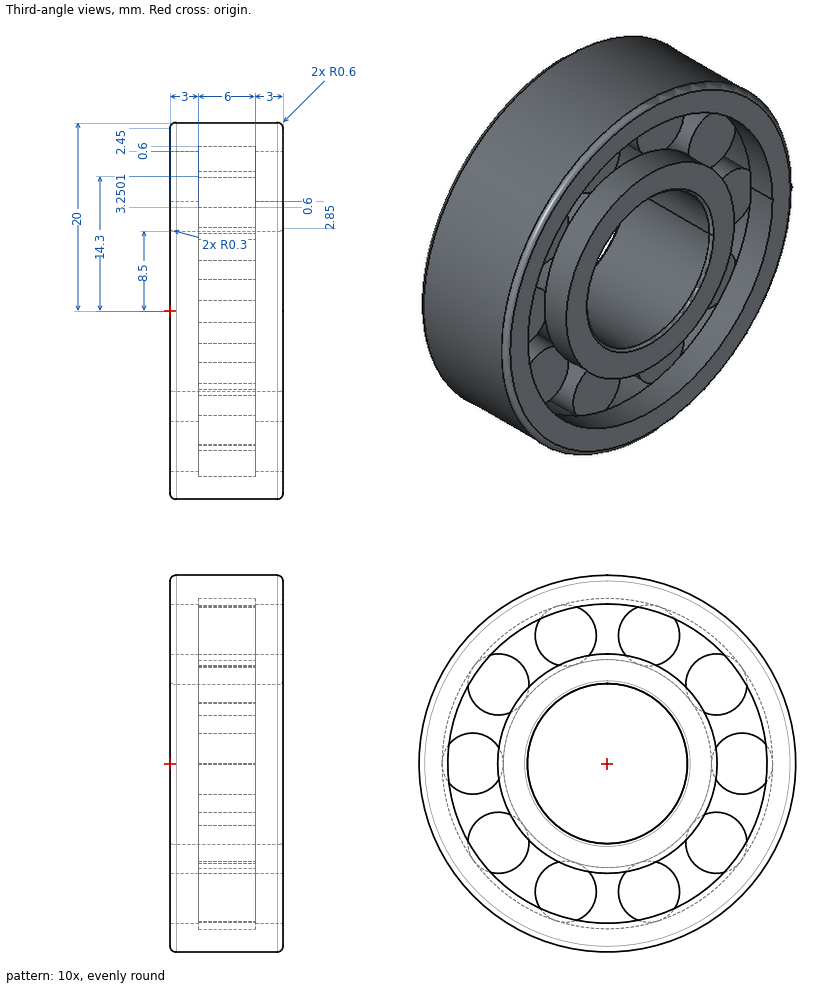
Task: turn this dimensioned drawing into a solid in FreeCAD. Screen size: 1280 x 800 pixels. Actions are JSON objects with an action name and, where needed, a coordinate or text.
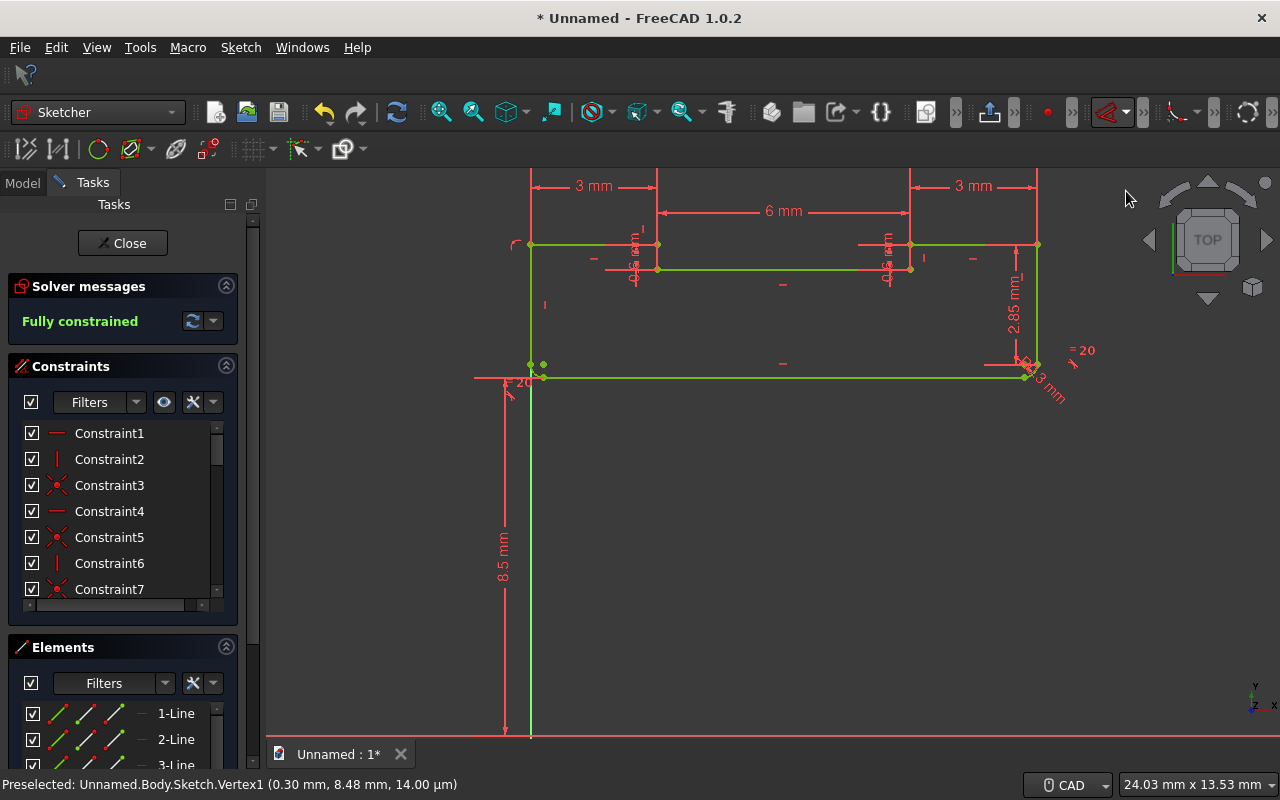
{"action": "left_click", "coordinate": [123, 243]}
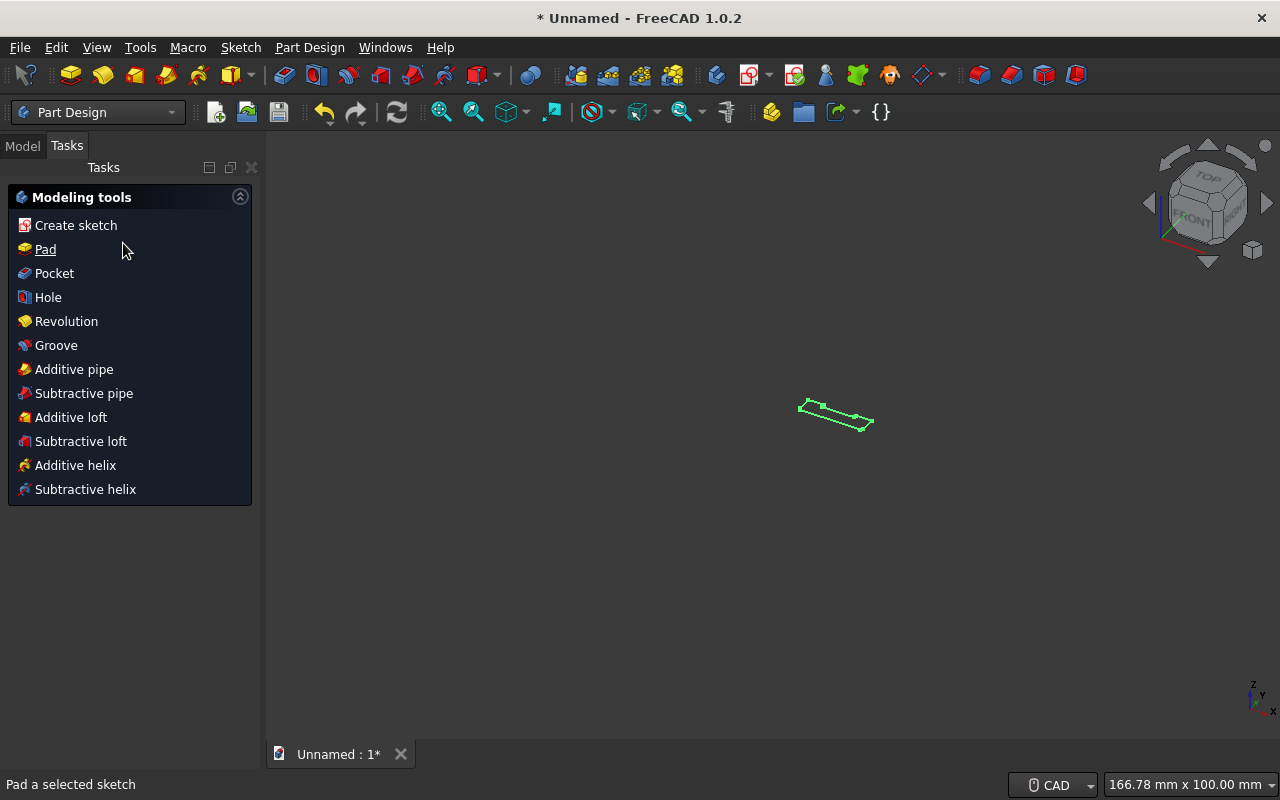
{"action": "left_click", "coordinate": [104, 76]}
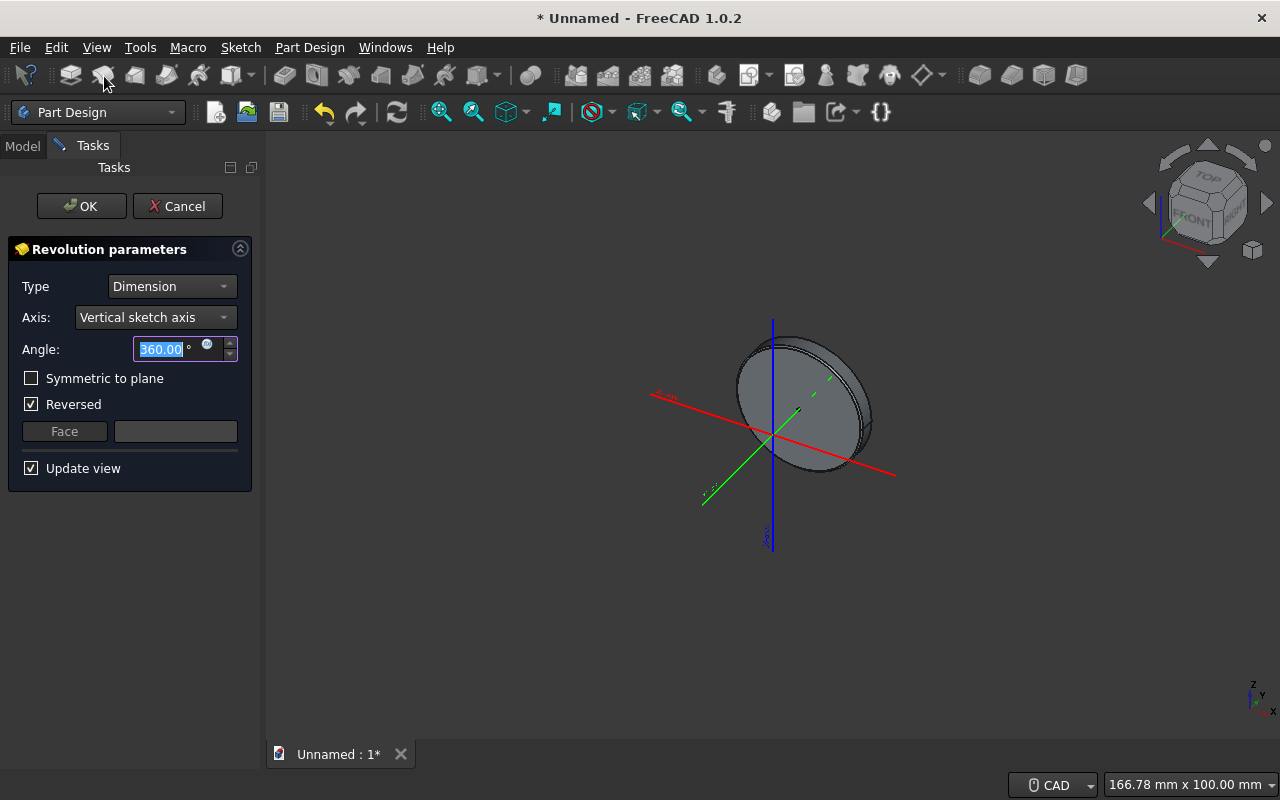
{"action": "left_click", "coordinate": [156, 318]}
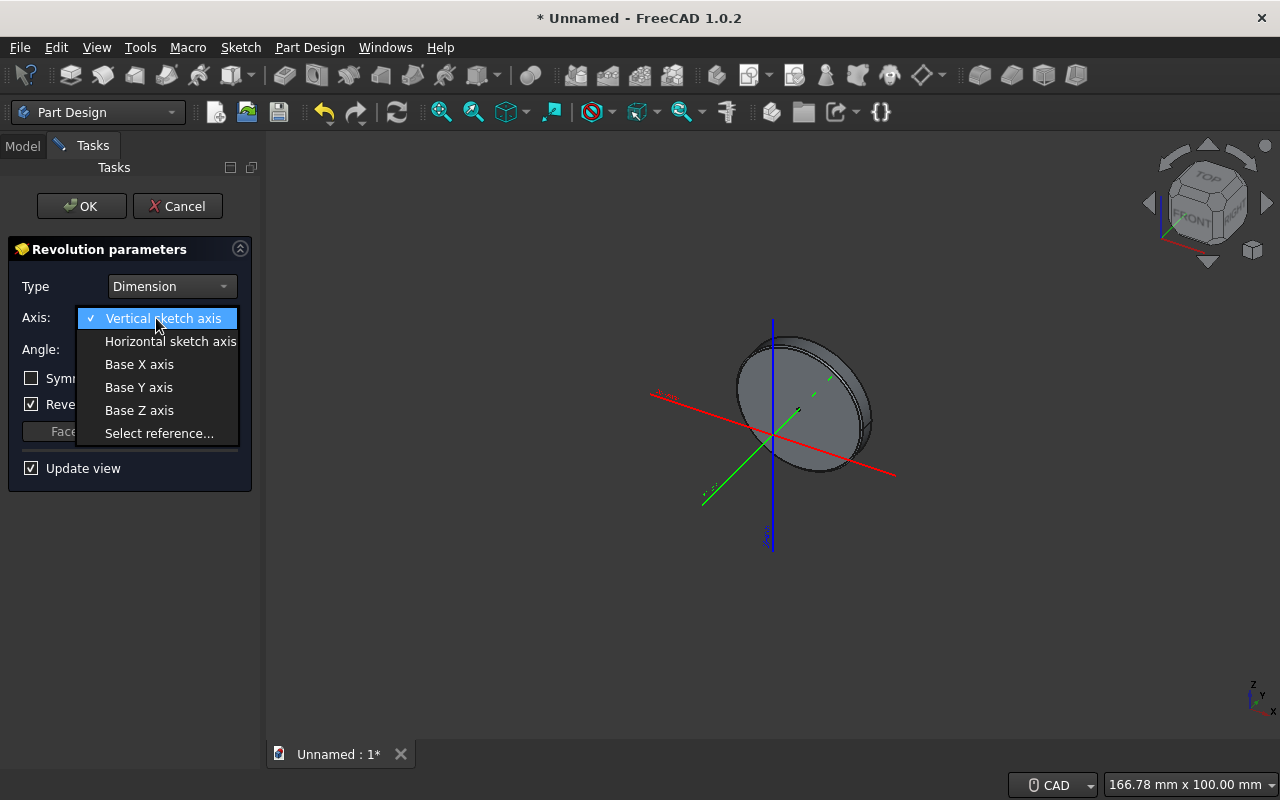
{"action": "left_click", "coordinate": [156, 342]}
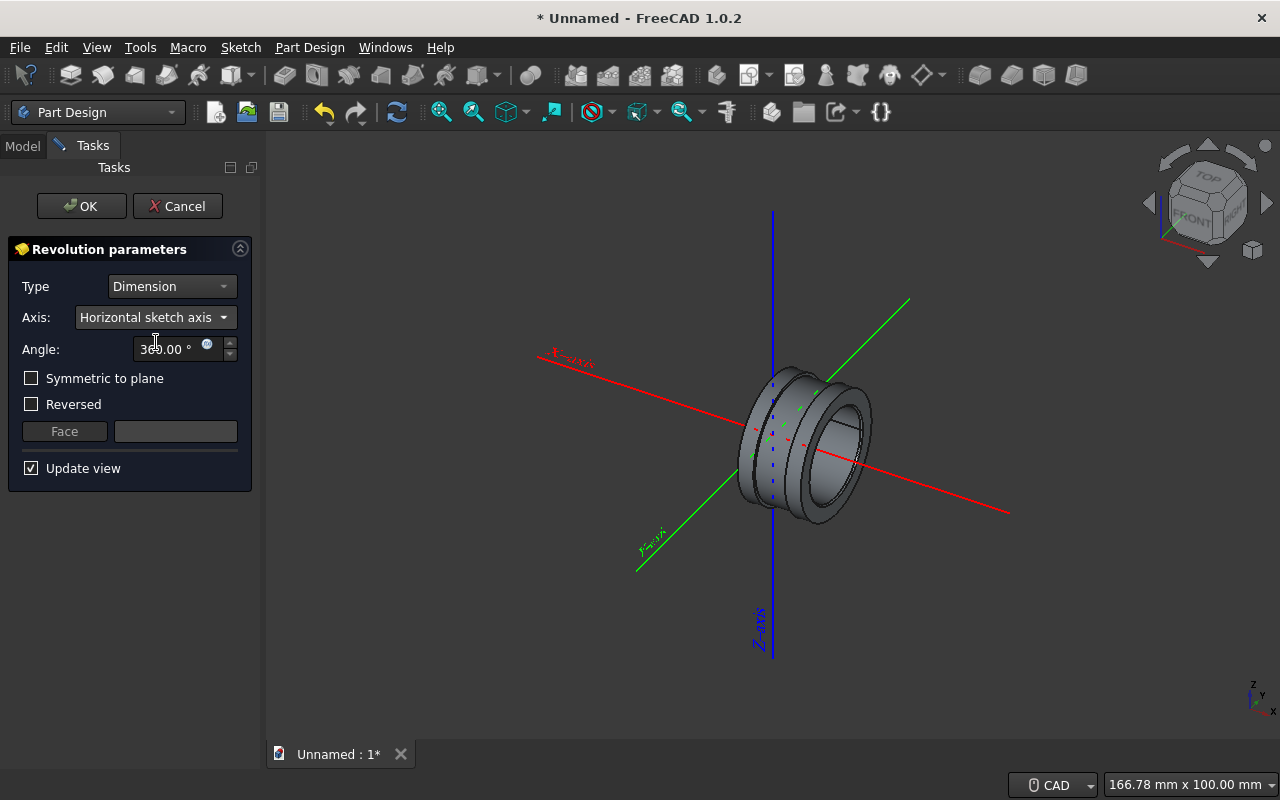
{"action": "left_click", "coordinate": [82, 206]}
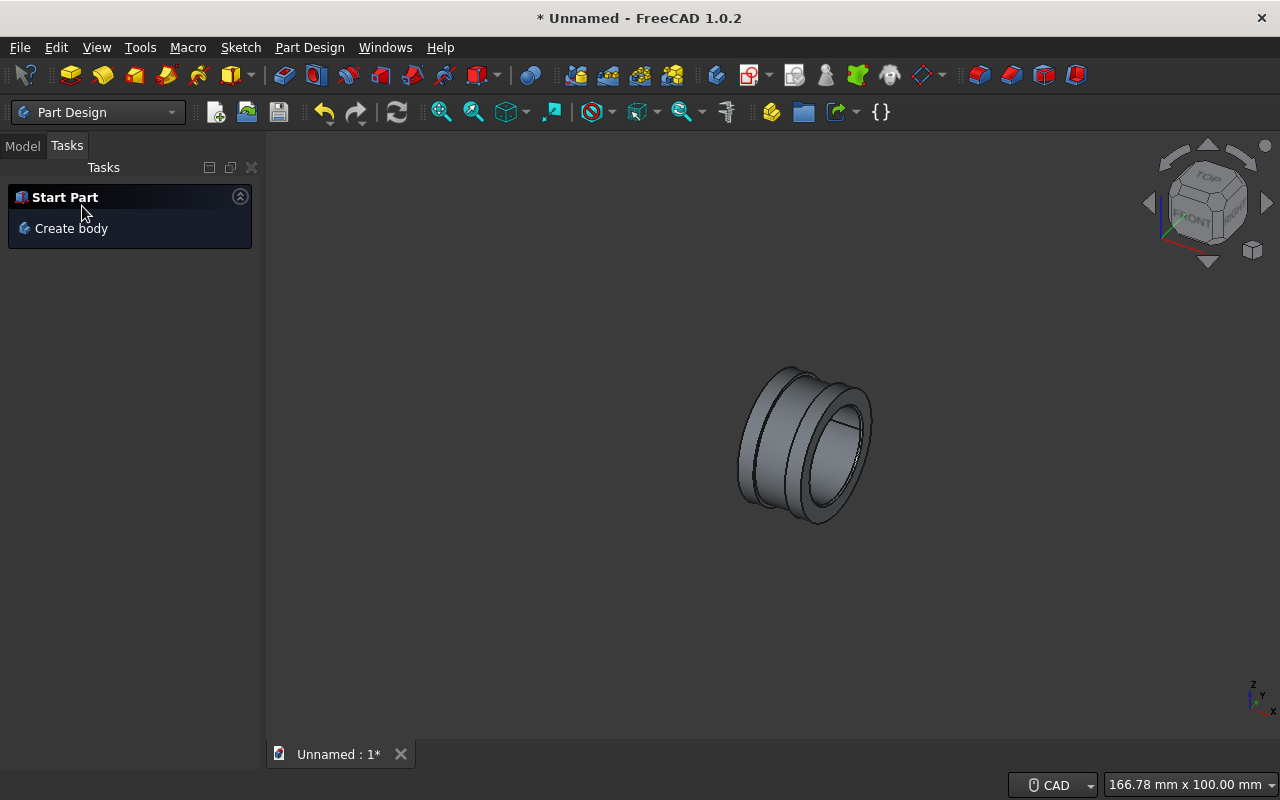
{"action": "left_click", "coordinate": [442, 112]}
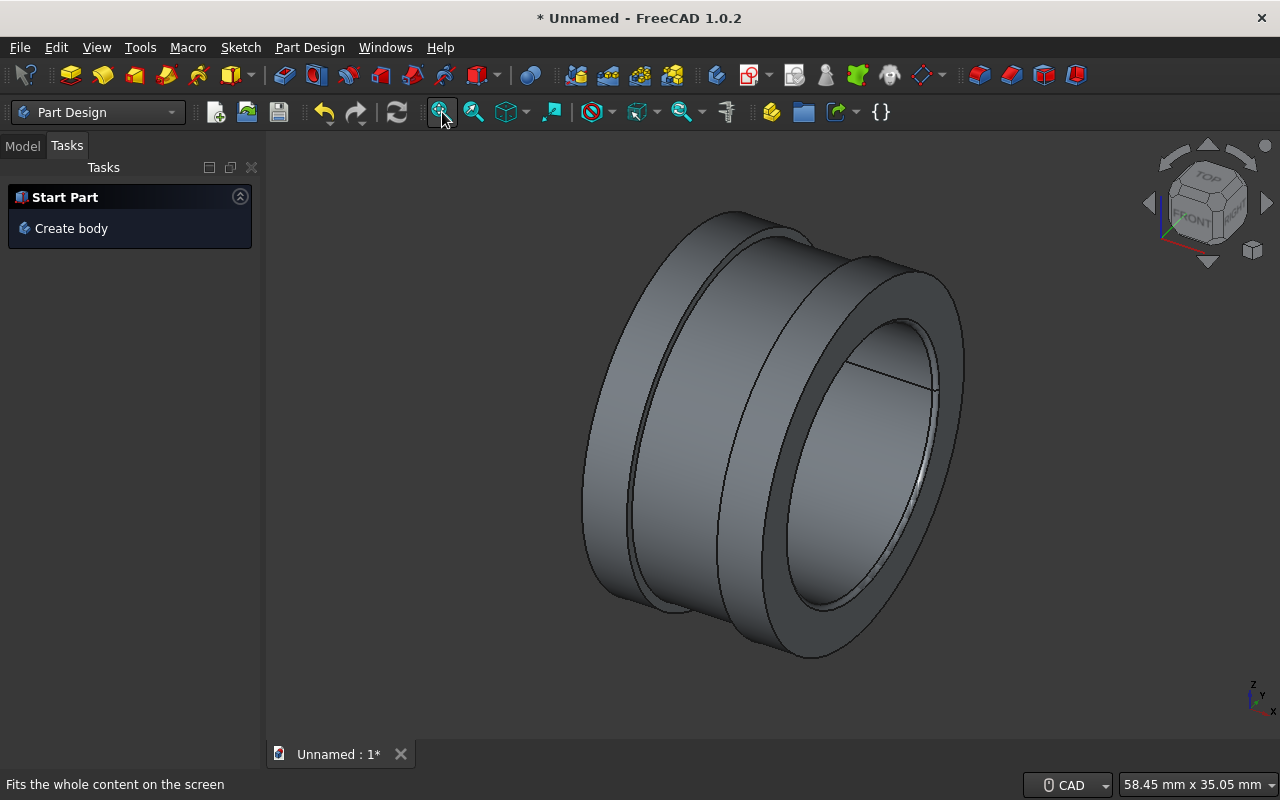
{"action": "left_click", "coordinate": [750, 76]}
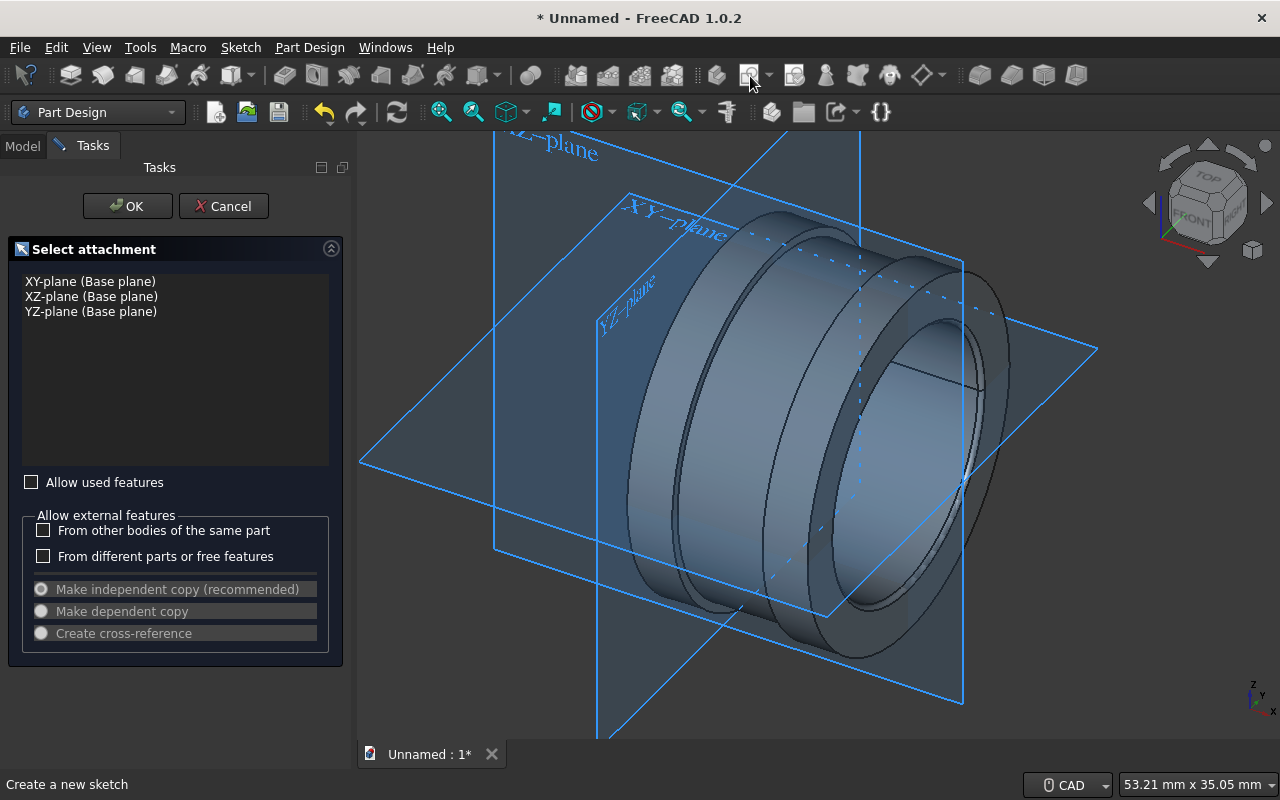
{"action": "left_click", "coordinate": [82, 282]}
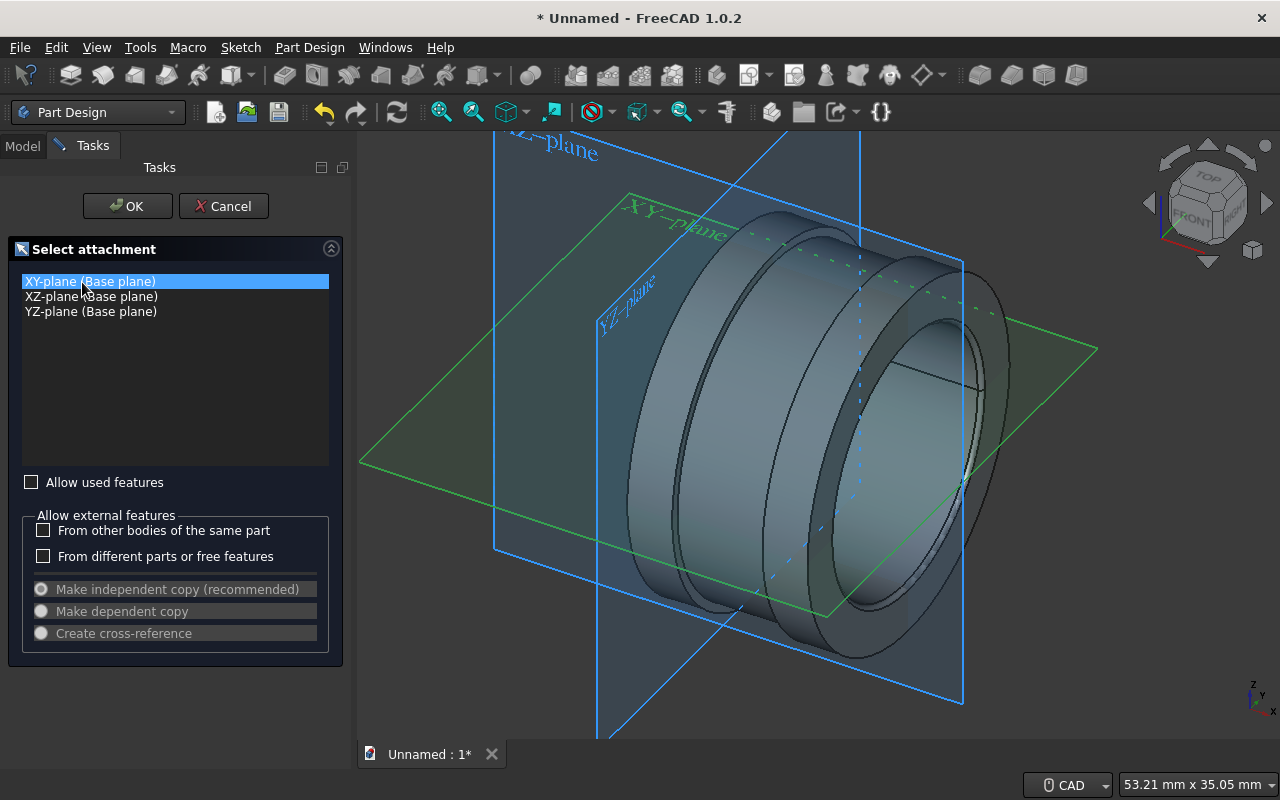
{"action": "left_click", "coordinate": [128, 206]}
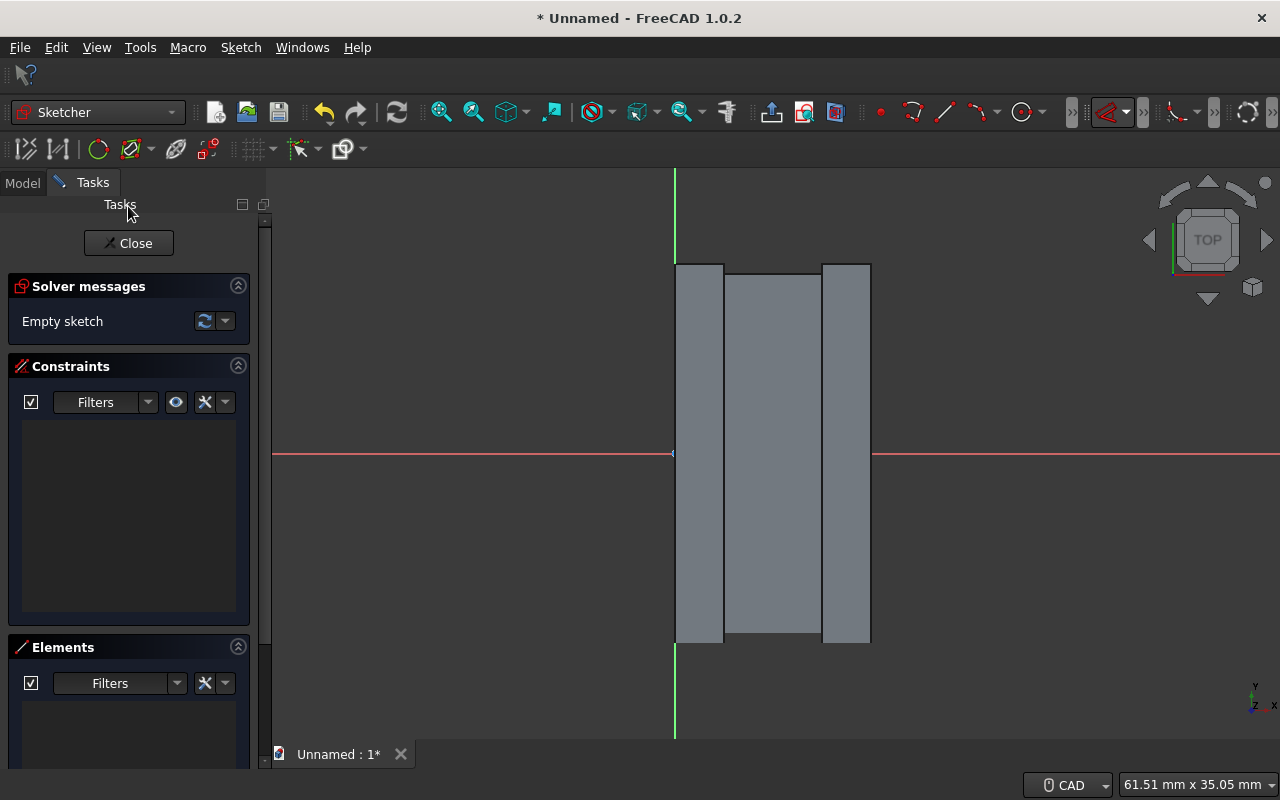
{"action": "left_click", "coordinate": [836, 112]}